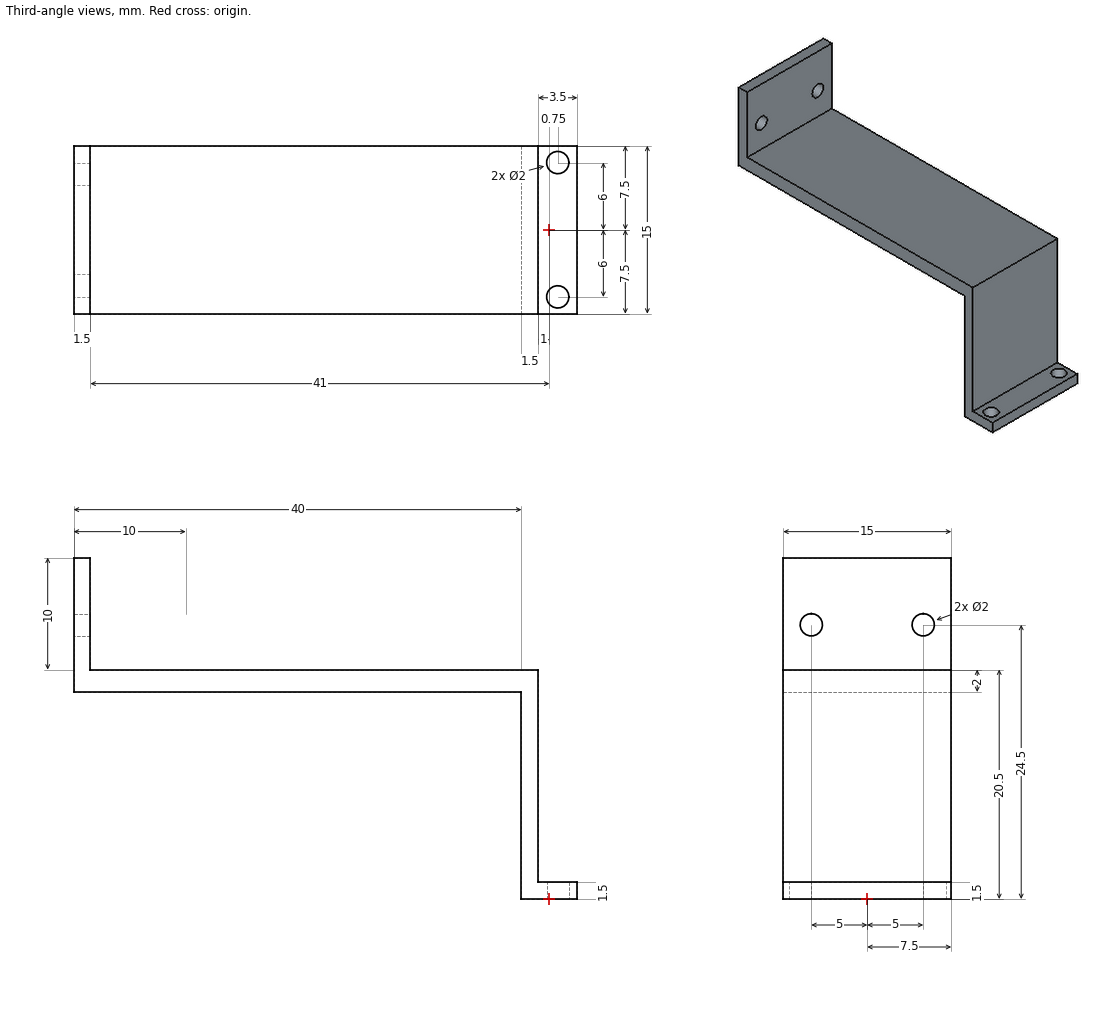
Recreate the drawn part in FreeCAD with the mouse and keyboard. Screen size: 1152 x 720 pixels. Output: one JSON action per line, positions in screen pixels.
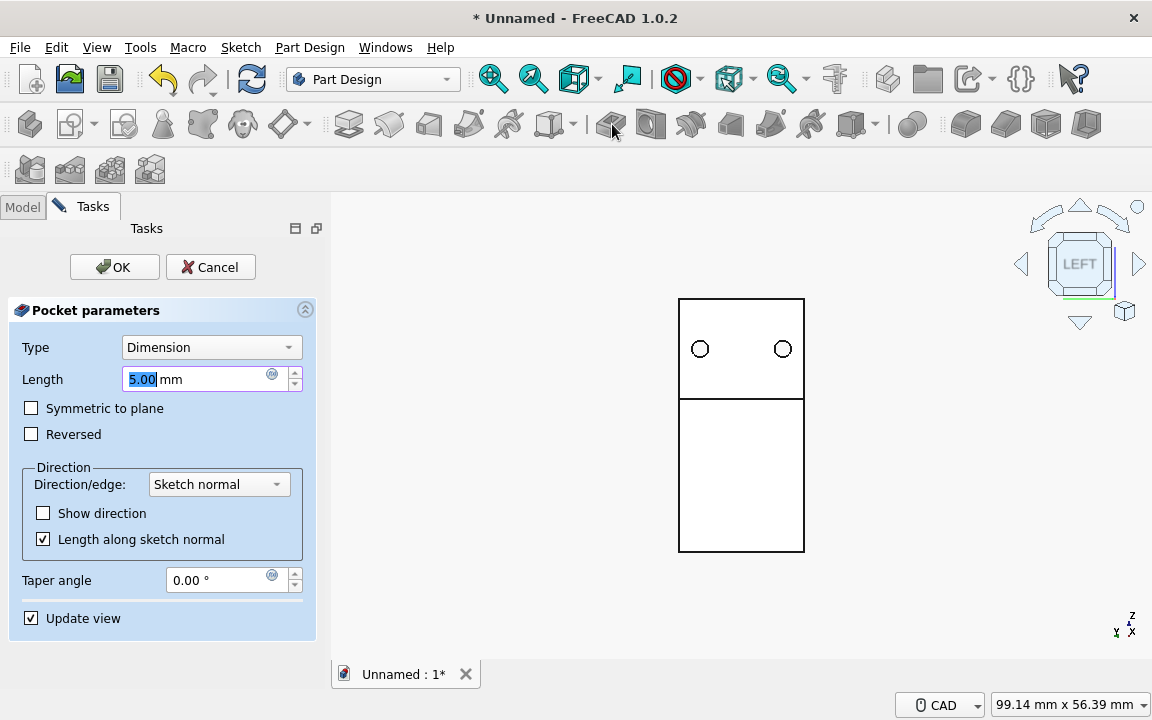
{"action": "type", "text": "10"}
{"action": "key", "text": "Tab"}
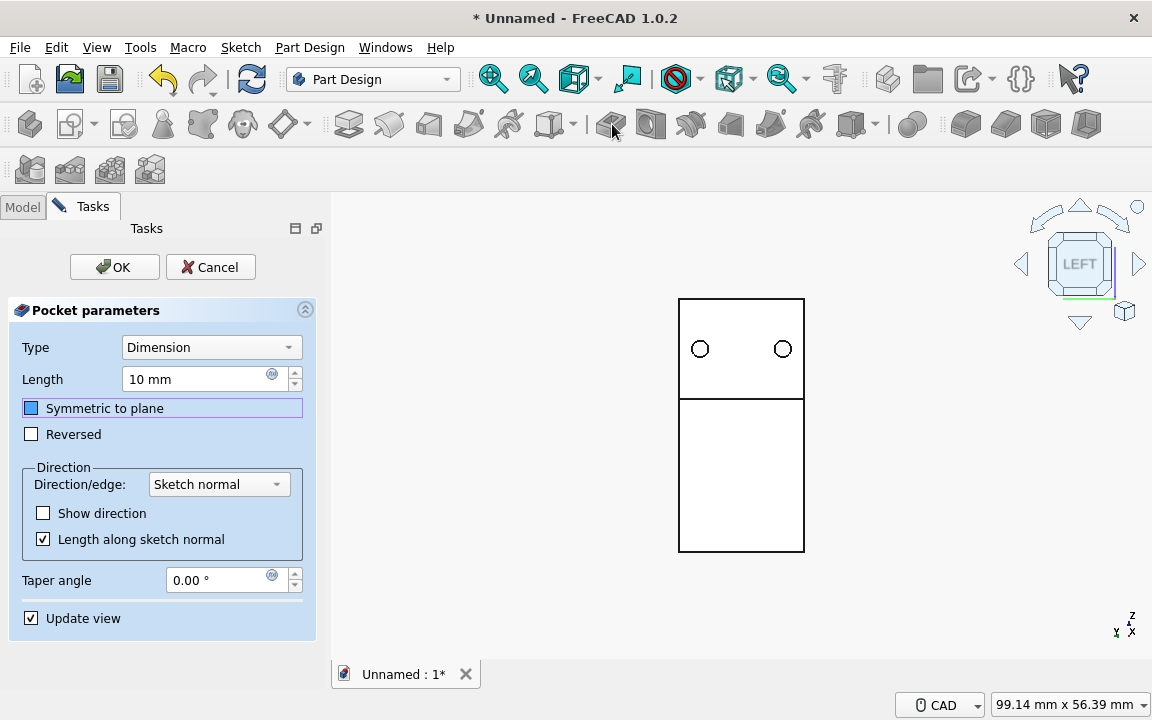
{"action": "left_click", "coordinate": [115, 267]}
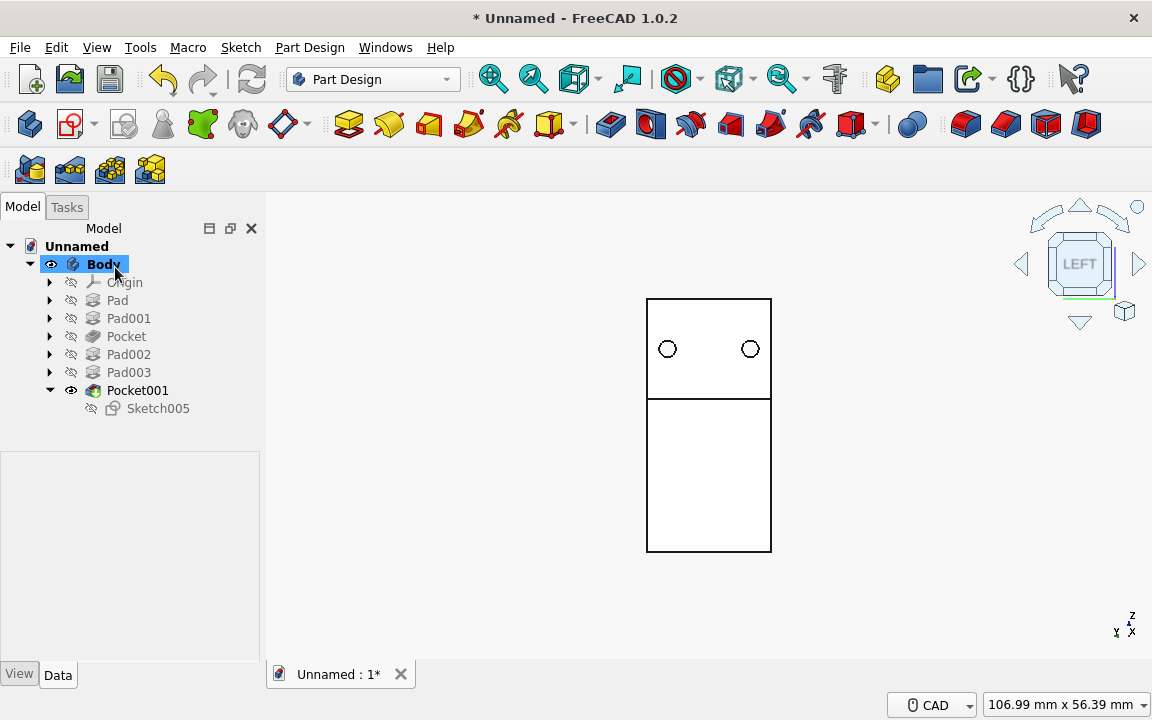
{"action": "key", "text": "0"}